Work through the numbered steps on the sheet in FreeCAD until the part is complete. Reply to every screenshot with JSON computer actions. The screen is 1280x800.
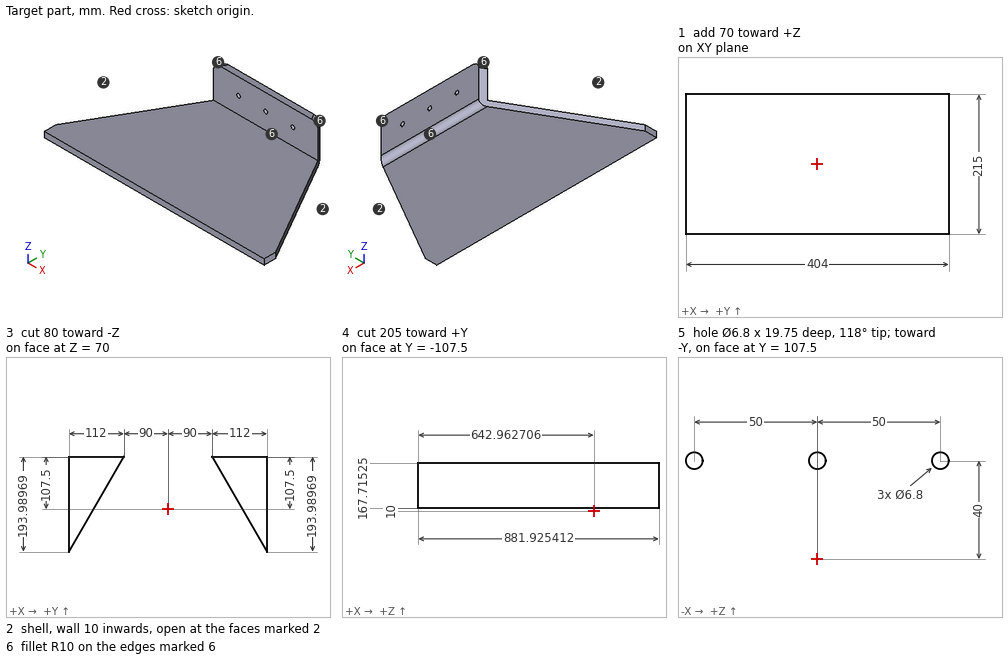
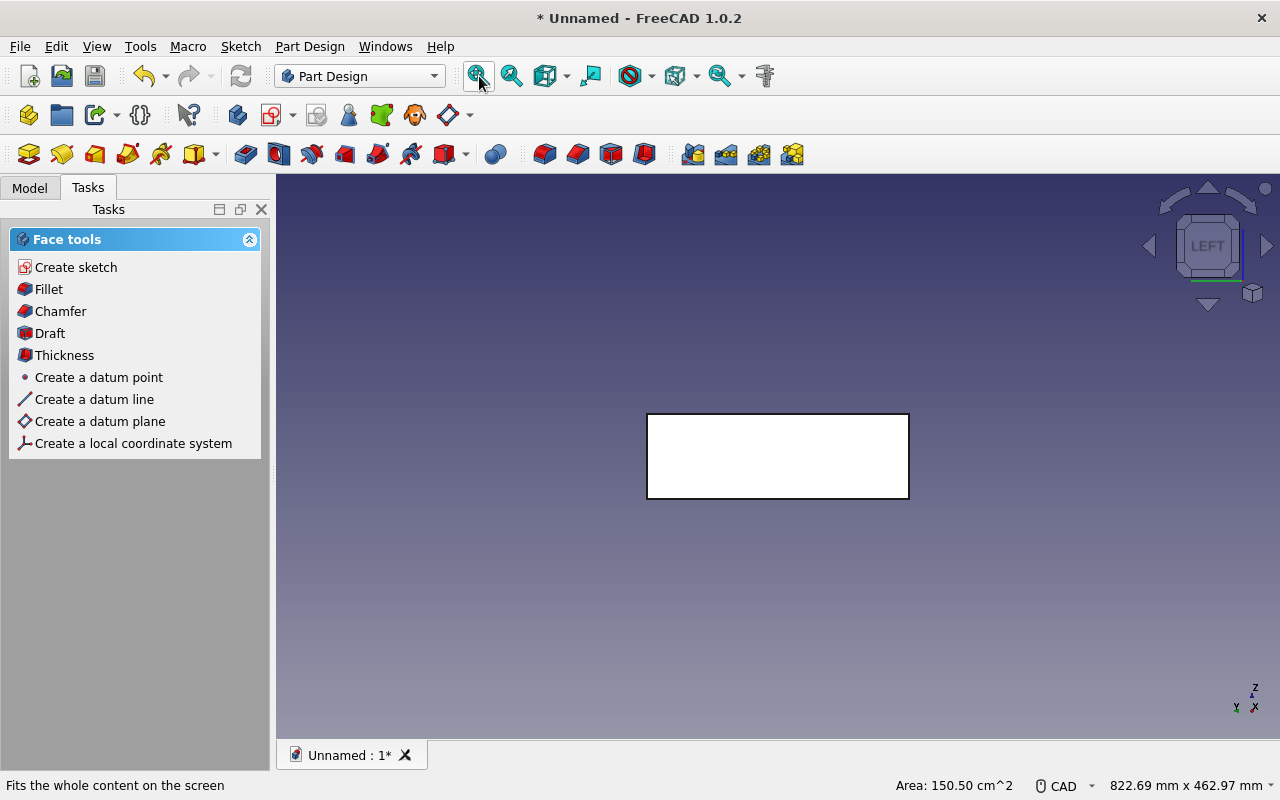
{"action": "left_click", "coordinate": [703, 455], "text": "ctrl"}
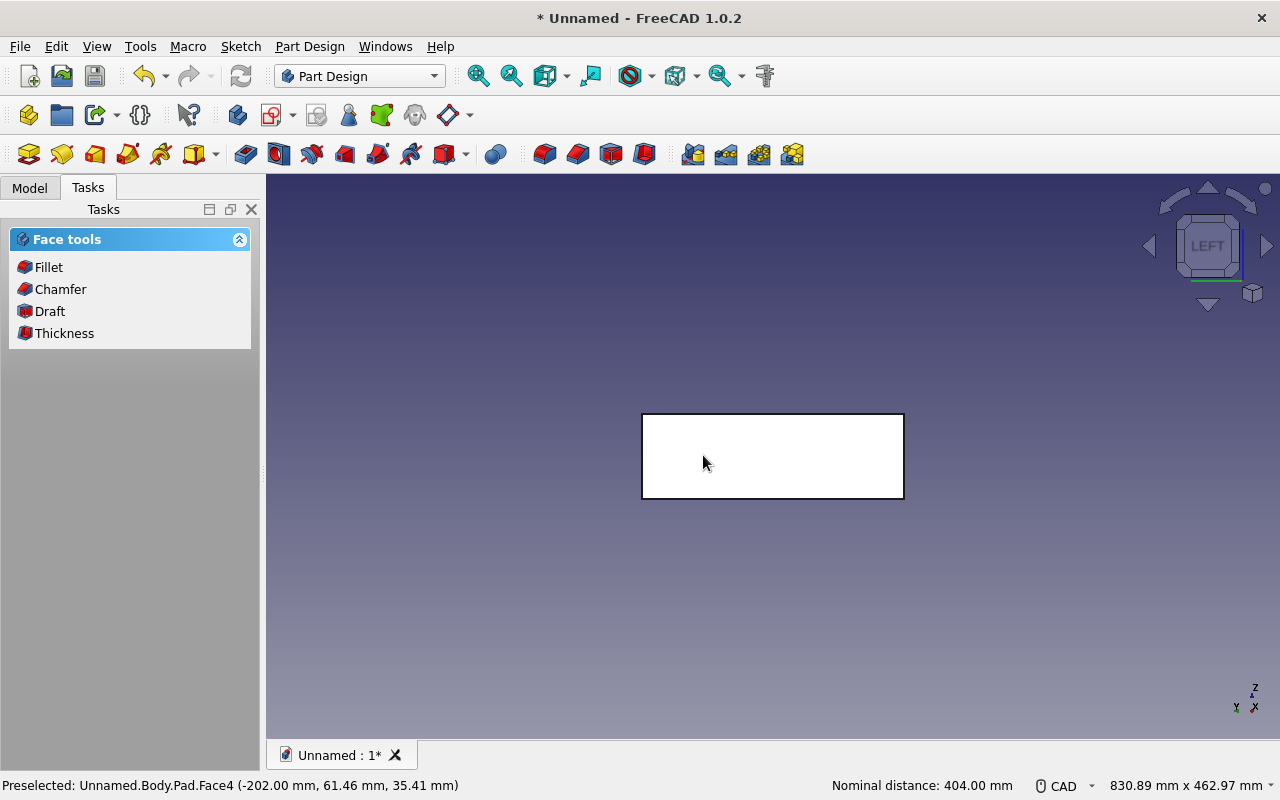
{"action": "left_click", "coordinate": [644, 154]}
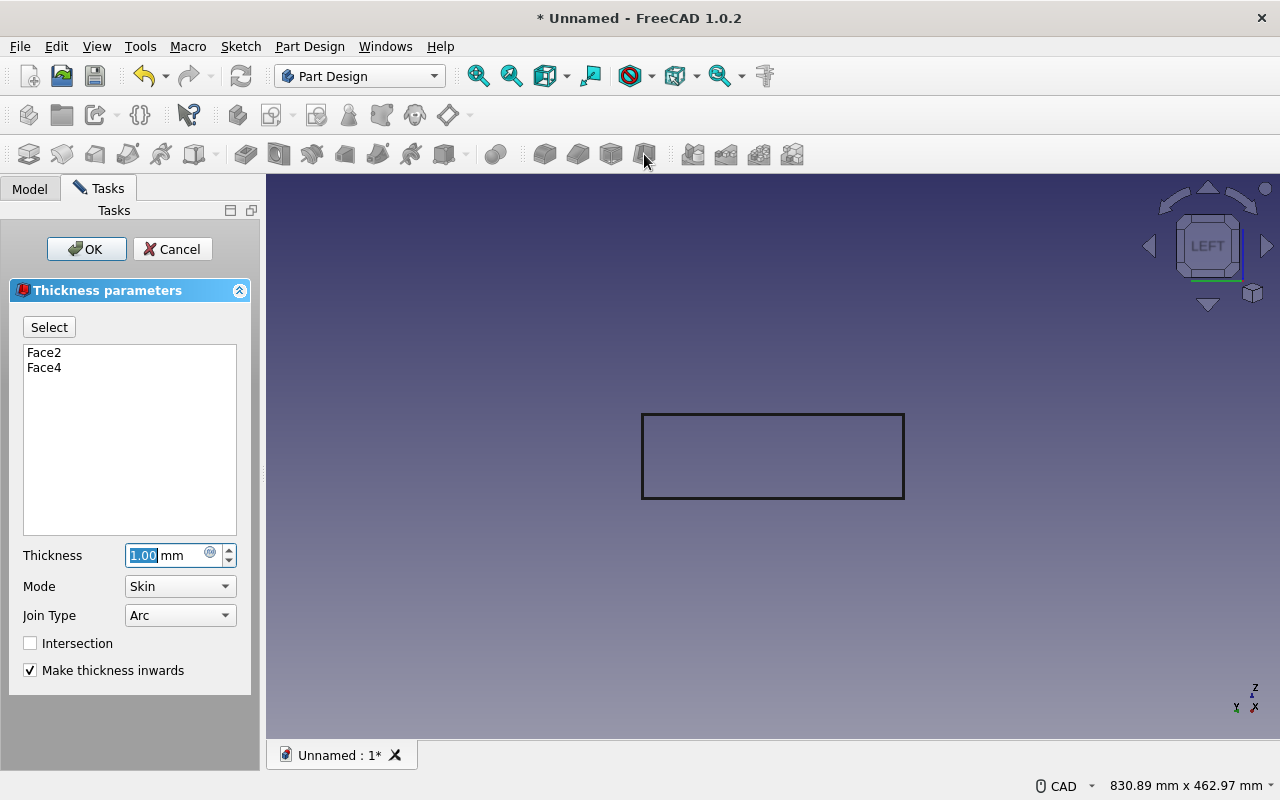
{"action": "type", "text": "10"}
{"action": "key", "text": "Tab"}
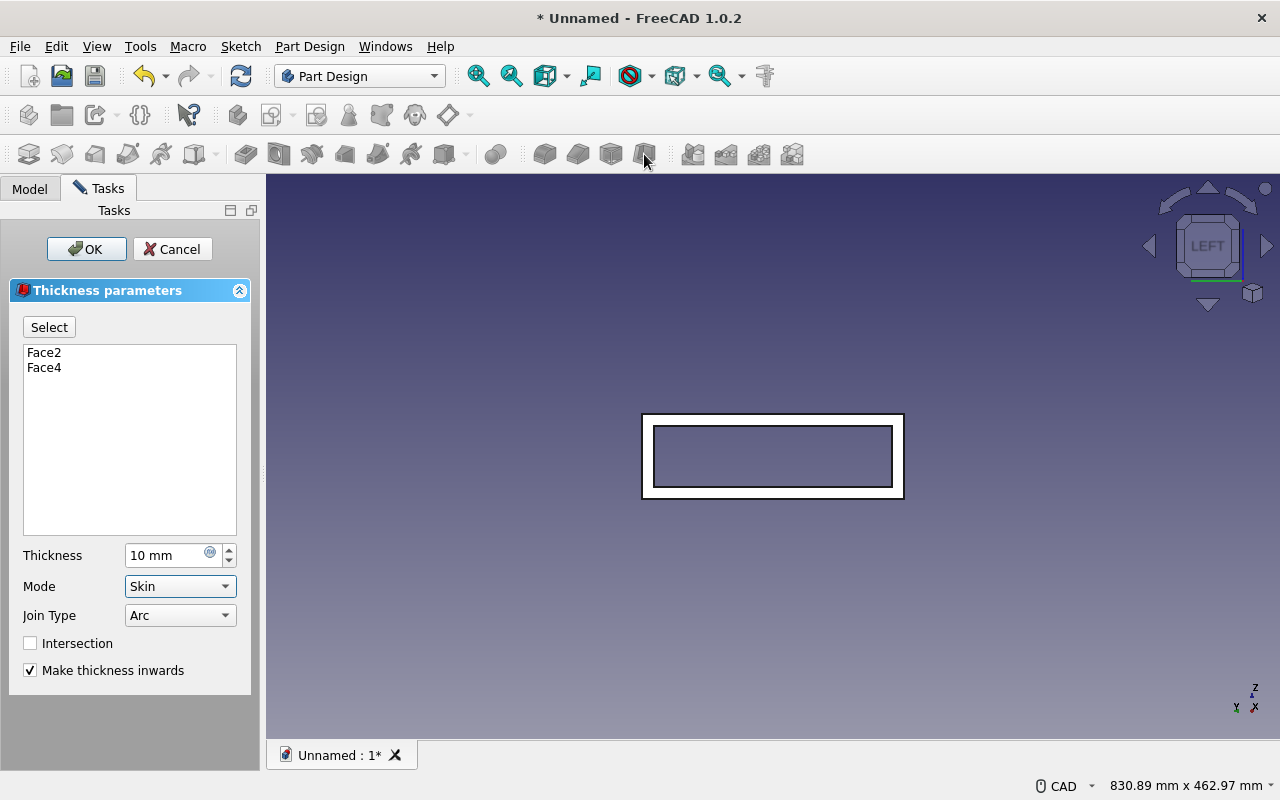
{"action": "left_click", "coordinate": [181, 616]}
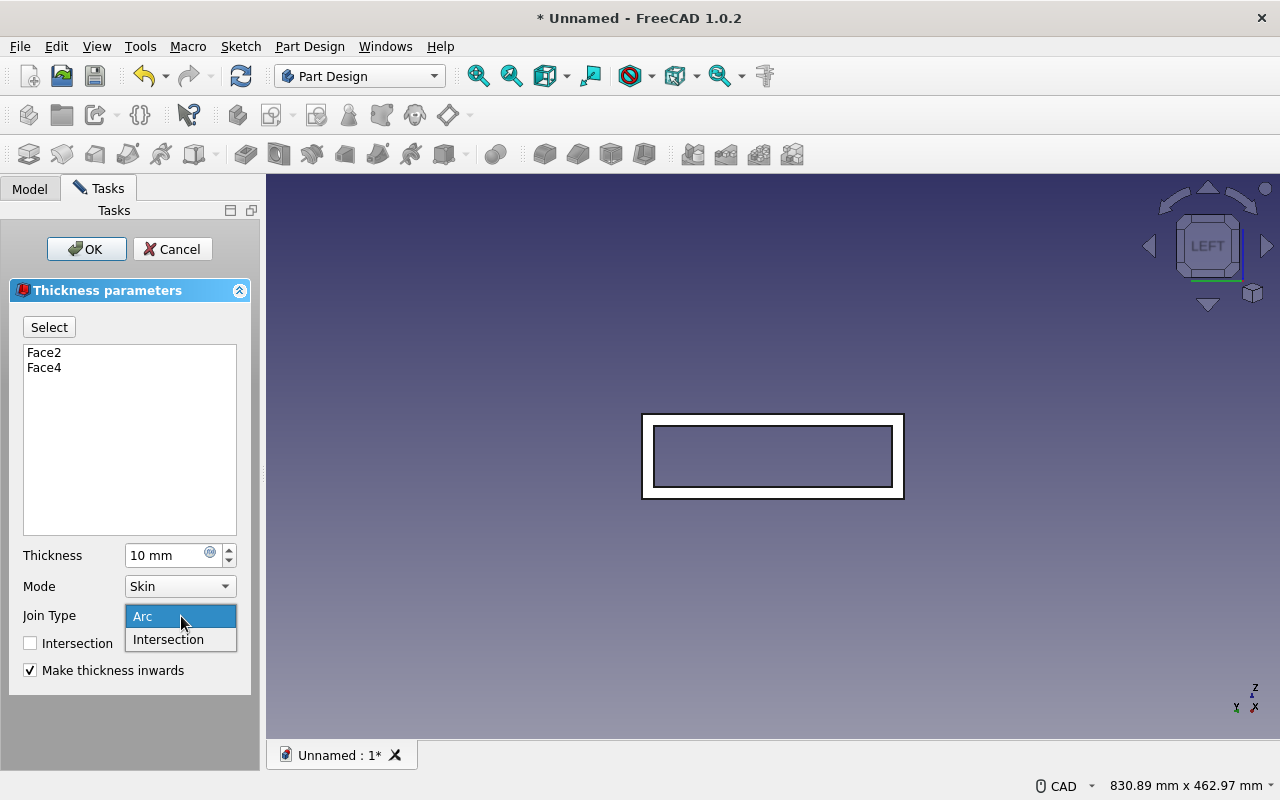
{"action": "left_click", "coordinate": [179, 640]}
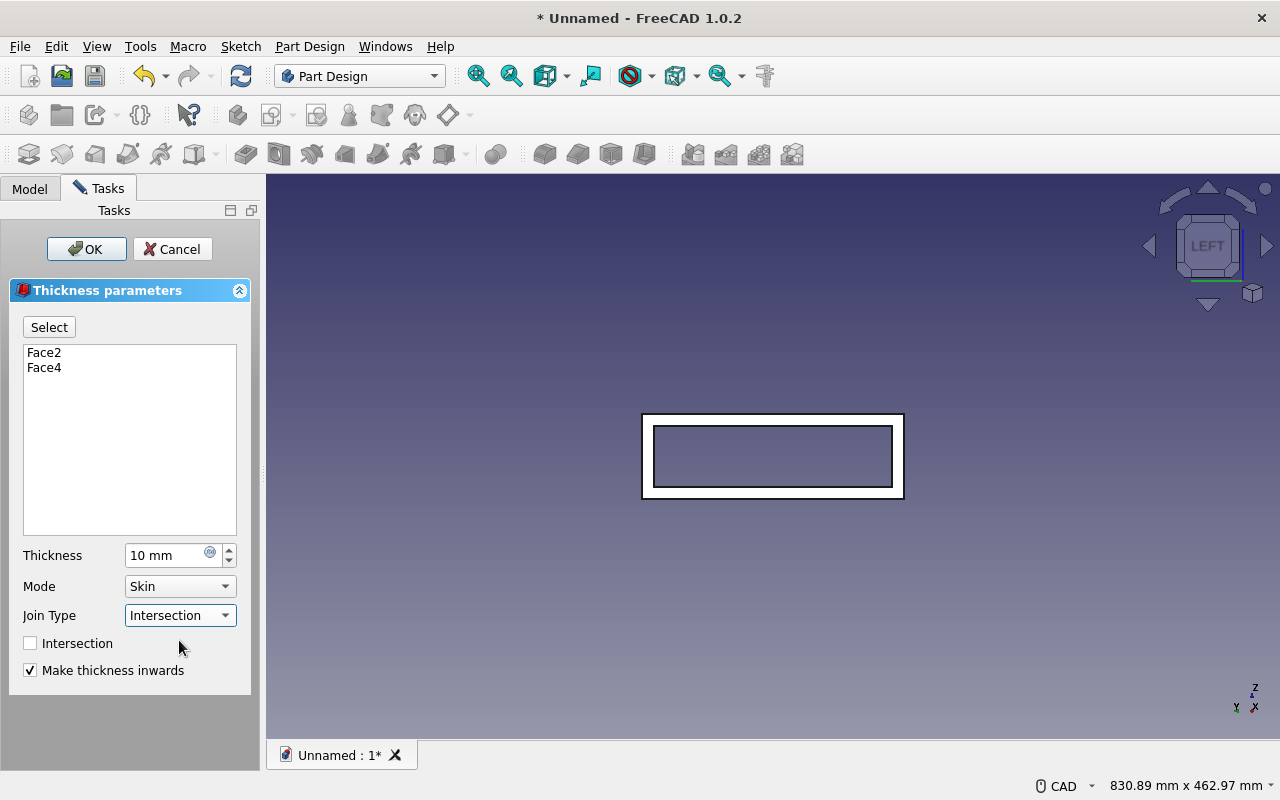
{"action": "left_click", "coordinate": [87, 249]}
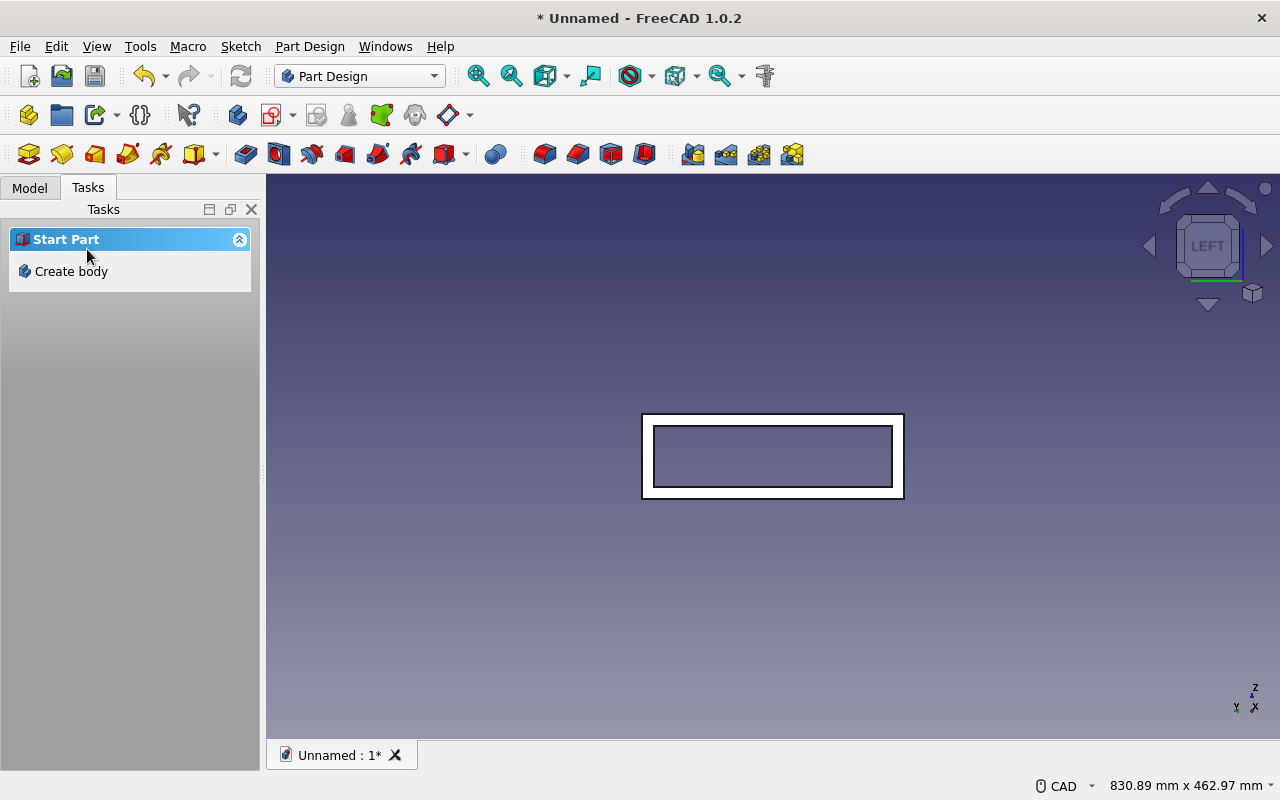
{"action": "left_click", "coordinate": [479, 76]}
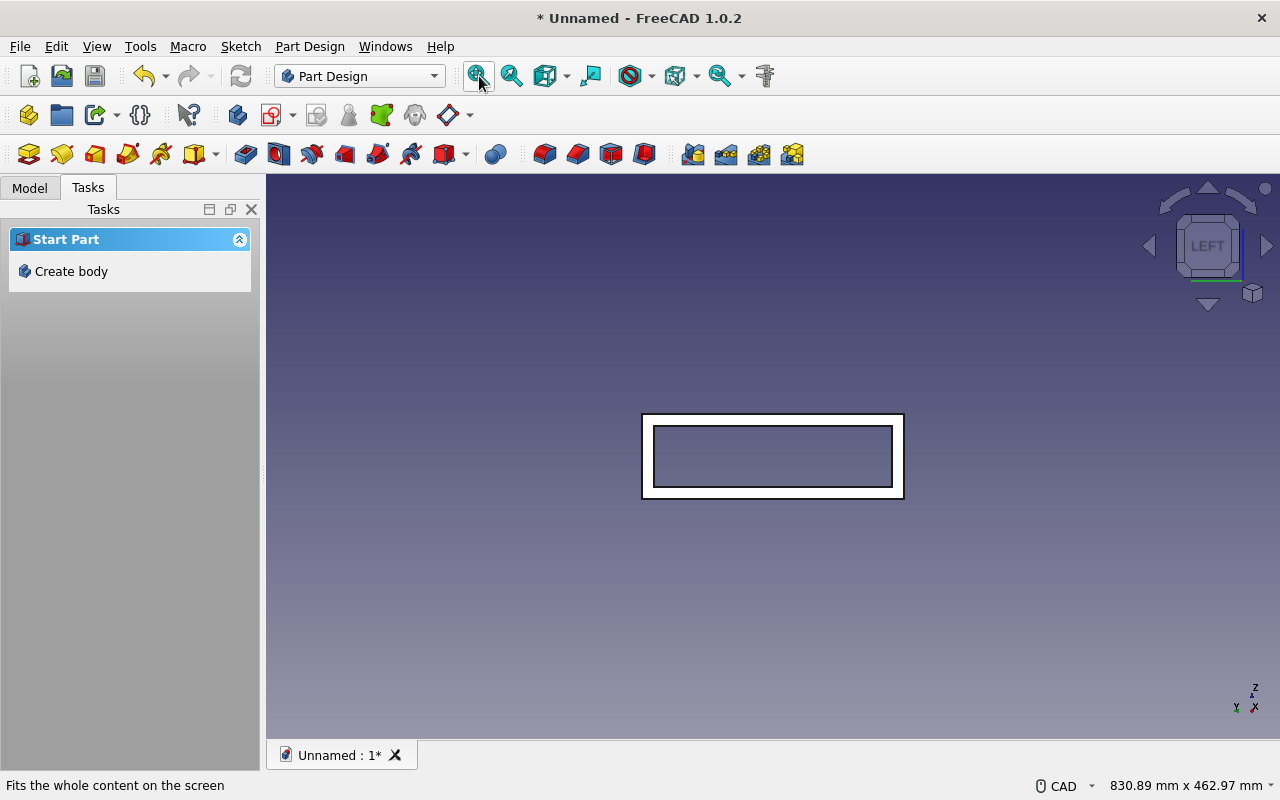
{"action": "key", "text": "0"}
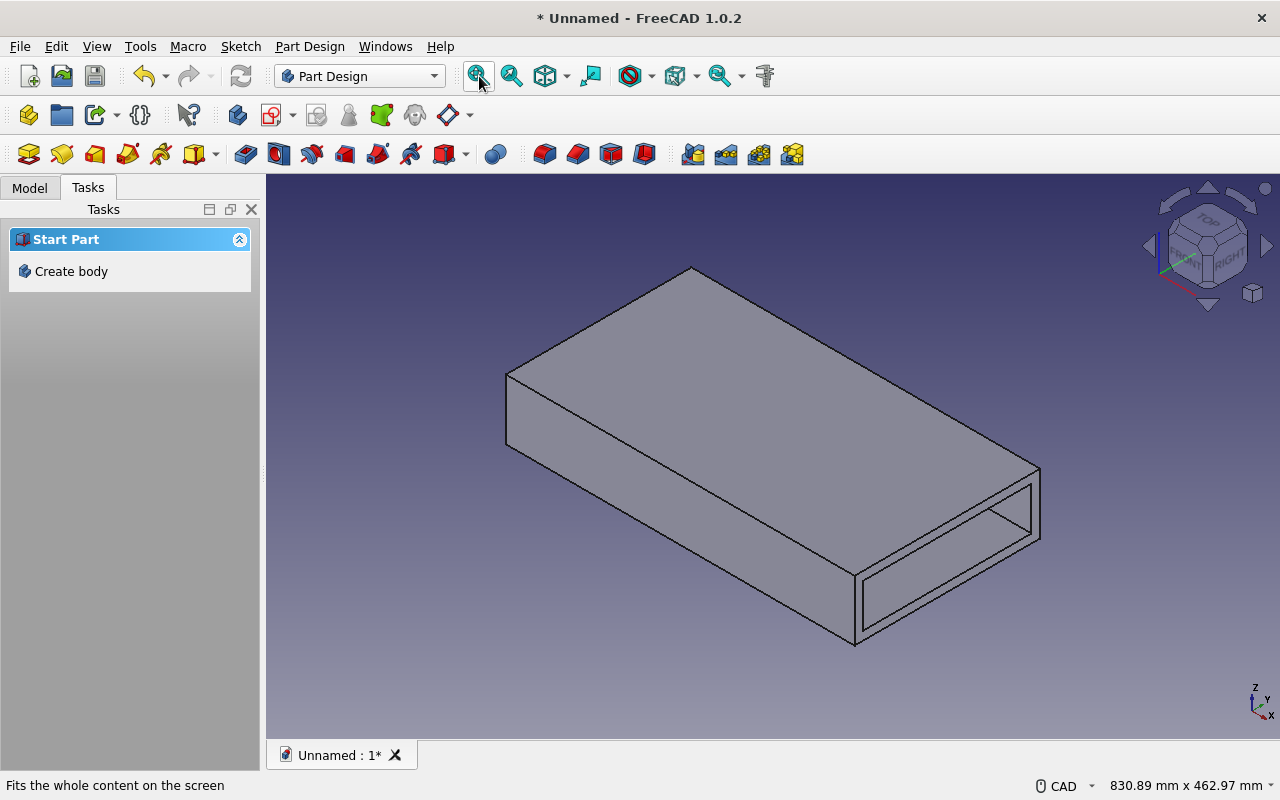
{"action": "left_click", "coordinate": [823, 449]}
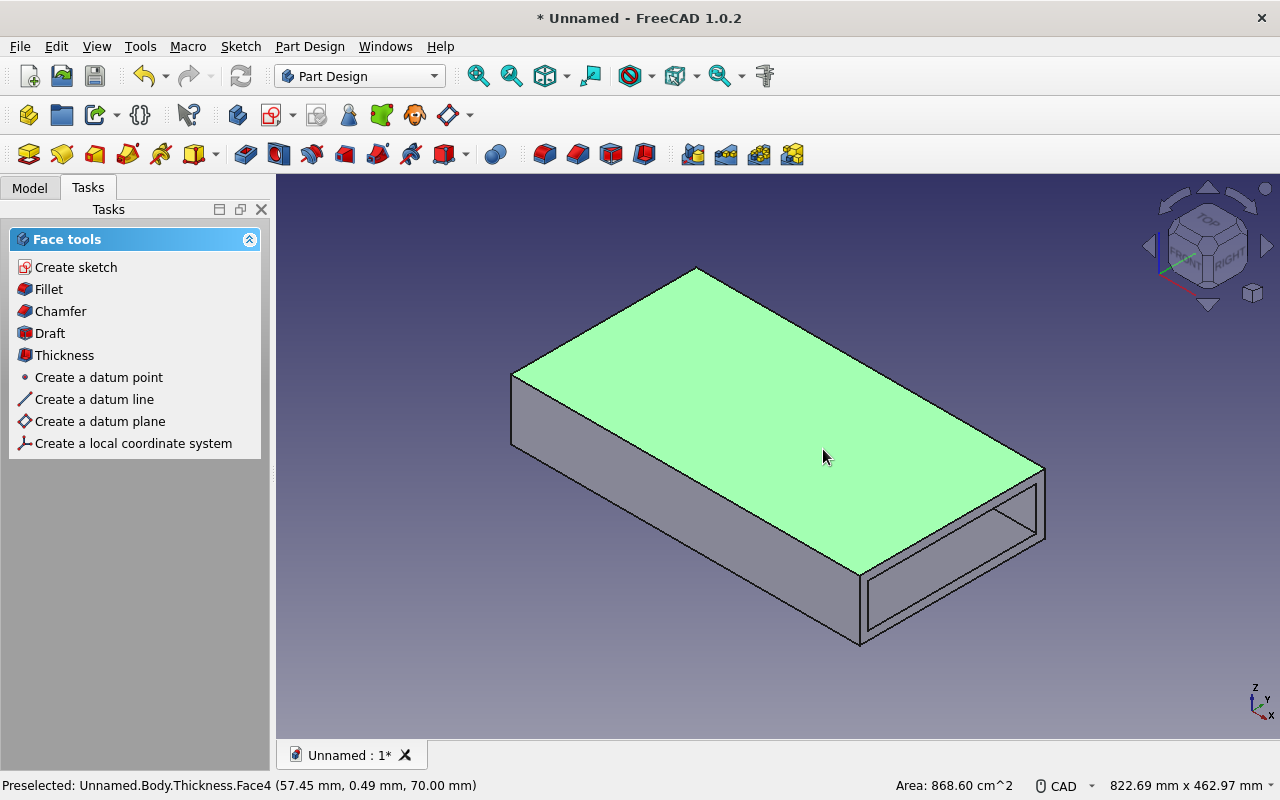
{"action": "left_click", "coordinate": [270, 116]}